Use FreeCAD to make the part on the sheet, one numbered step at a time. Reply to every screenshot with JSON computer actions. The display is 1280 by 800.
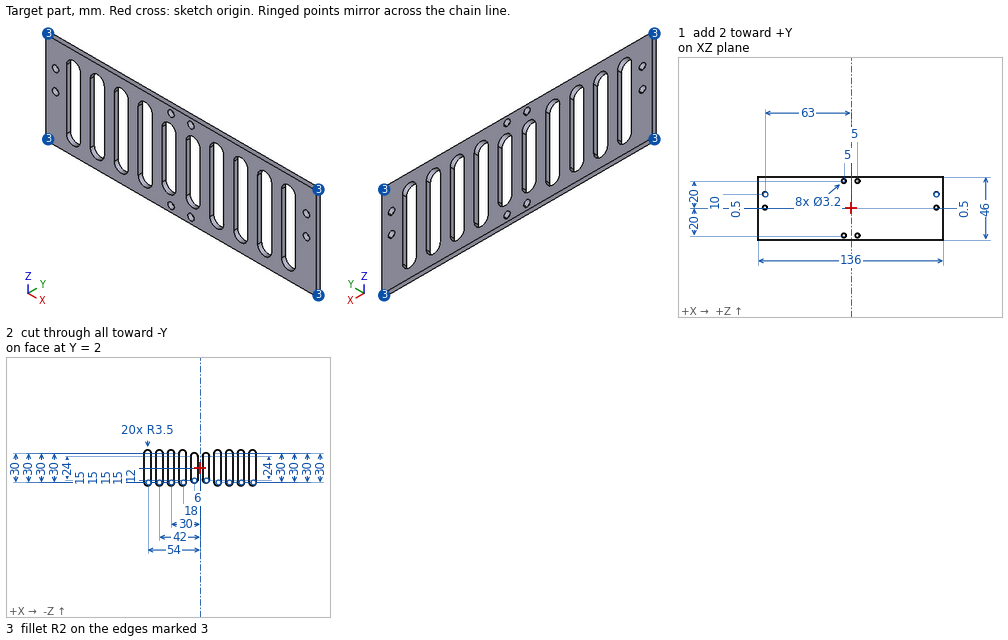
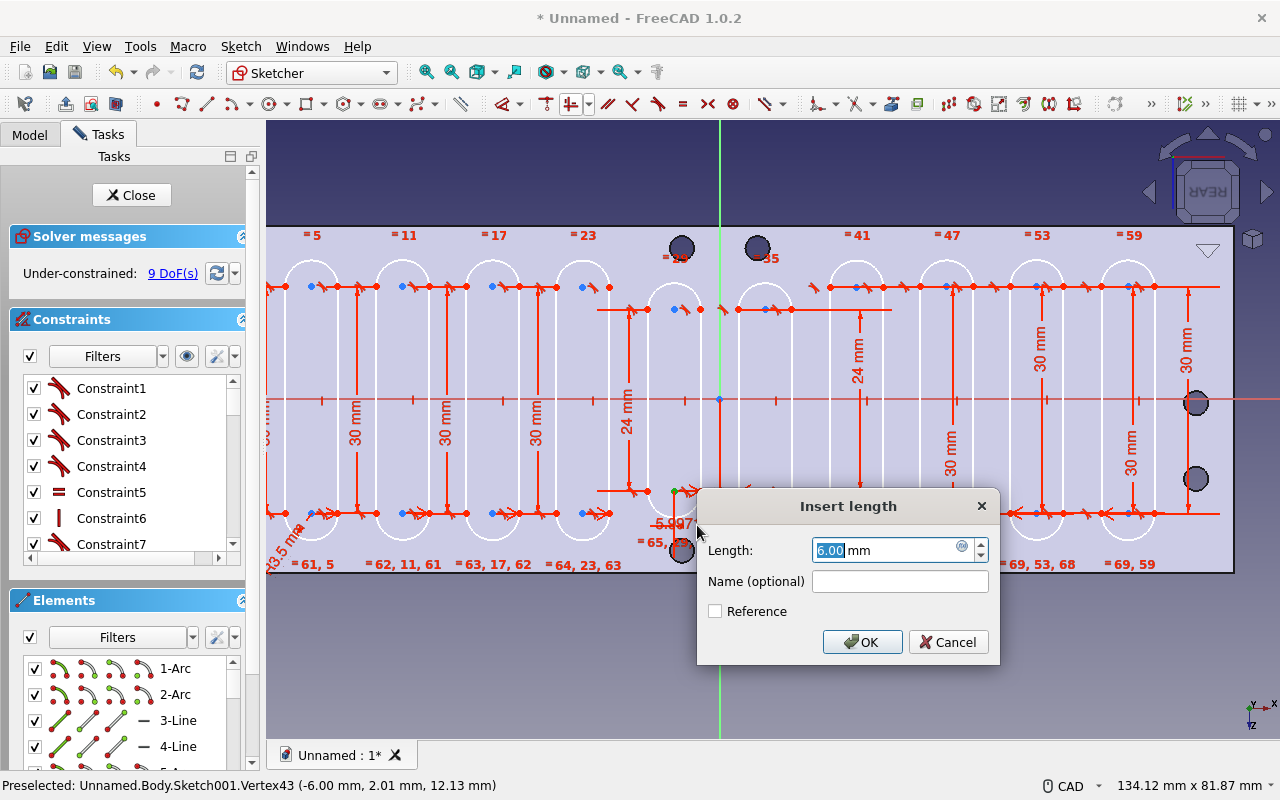
{"action": "type", "text": "6"}
{"action": "key", "text": "Return"}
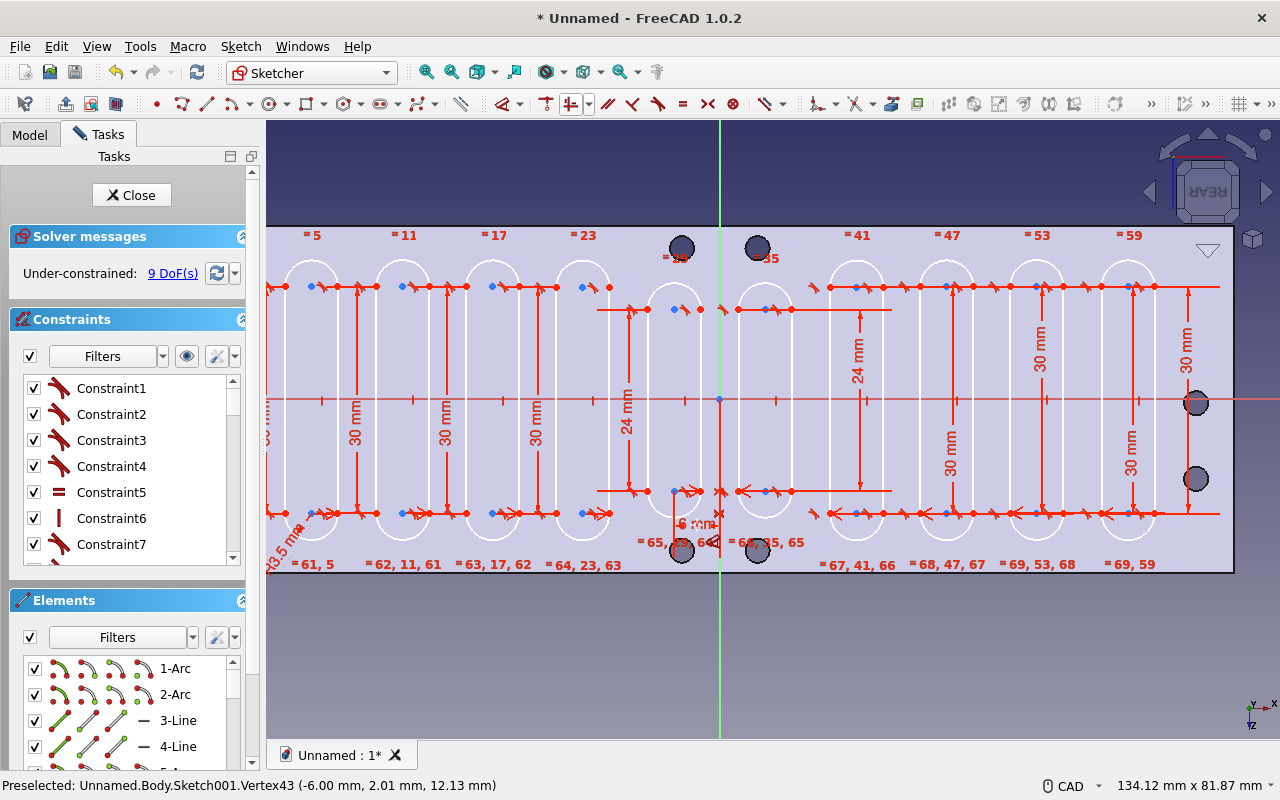
{"action": "scroll", "coordinate": [673, 491], "scroll_direction": "down", "scroll_amount": 2}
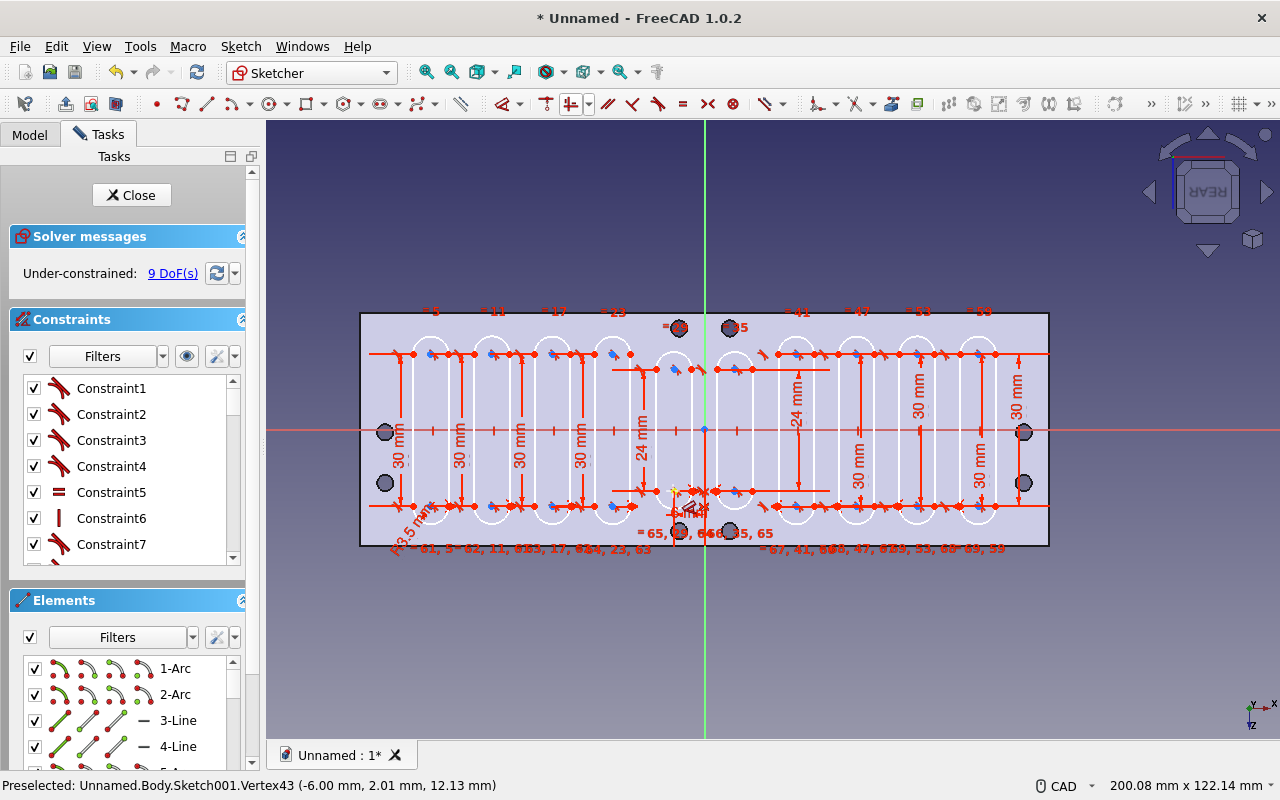
{"action": "left_click", "coordinate": [413, 506]}
{"action": "left_click", "coordinate": [379, 468]}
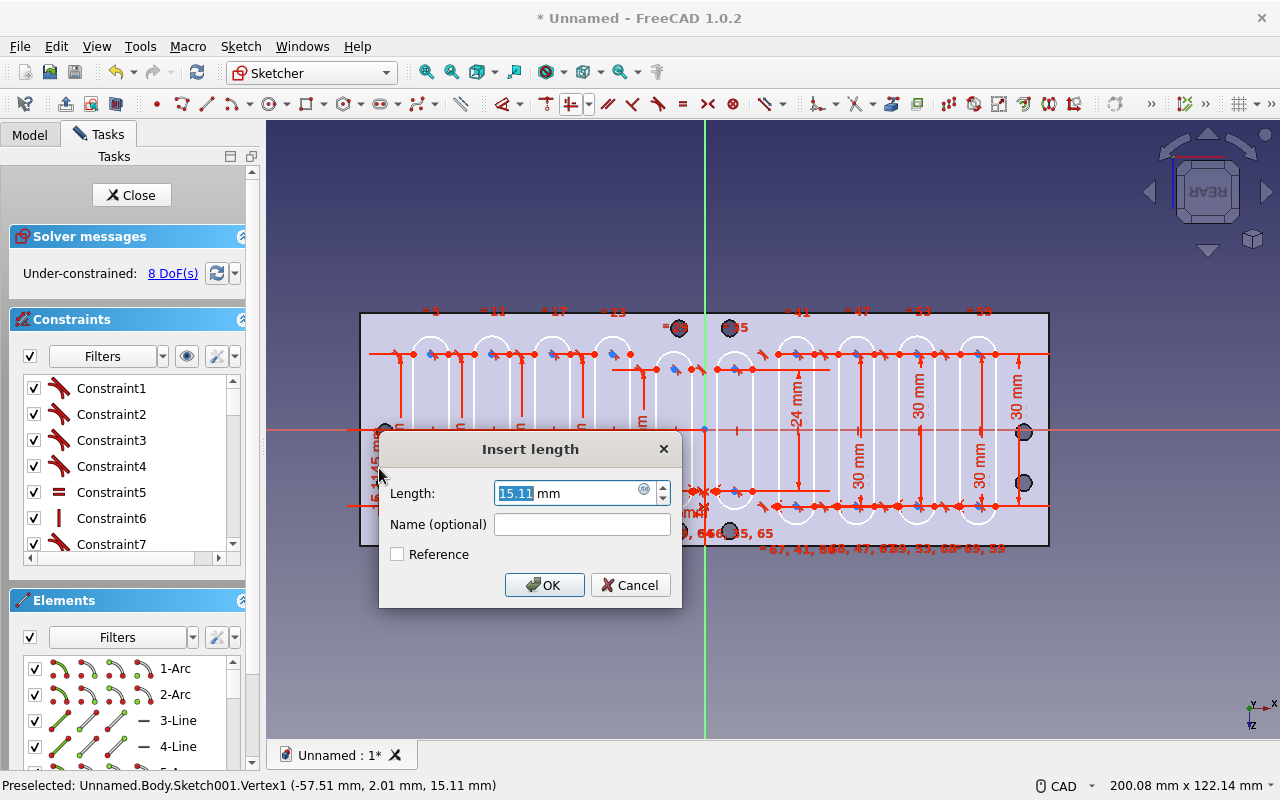
{"action": "type", "text": "15"}
{"action": "key", "text": "Return"}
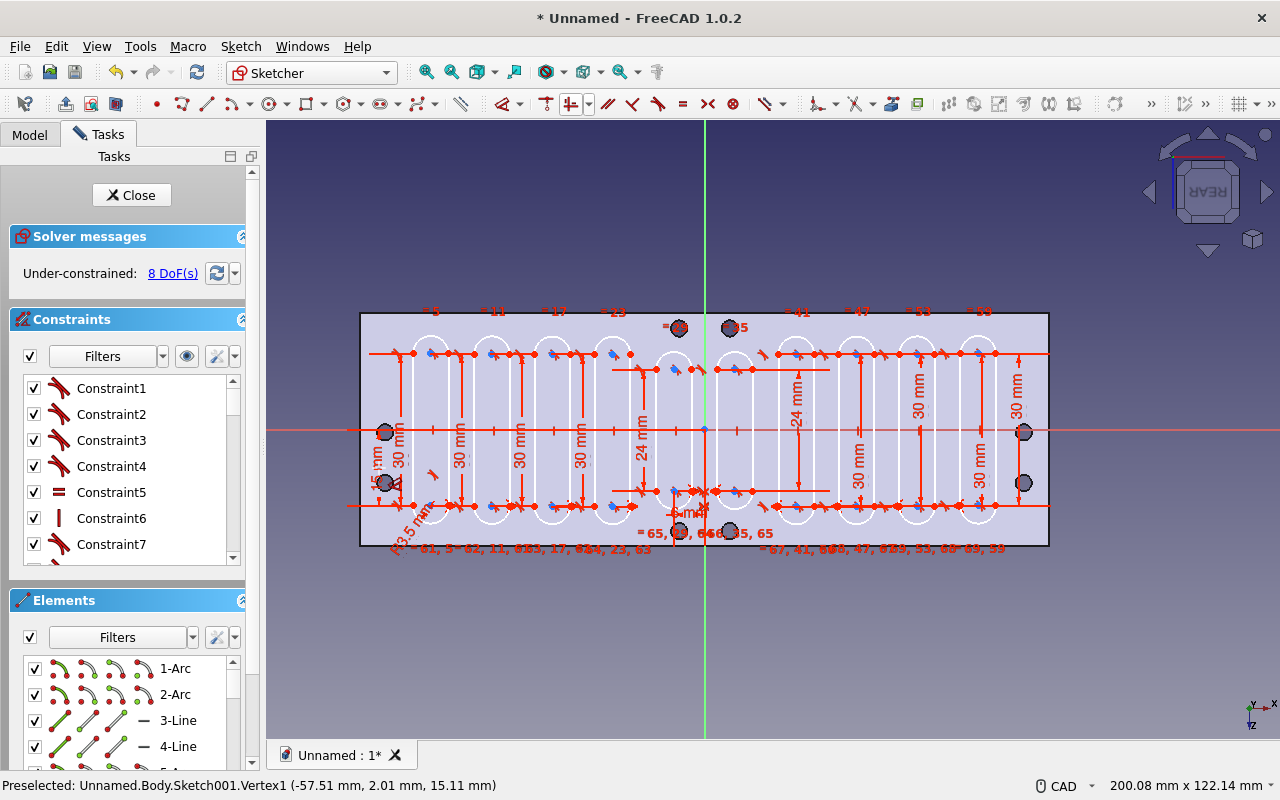
{"action": "left_click", "coordinate": [474, 506]}
{"action": "left_click", "coordinate": [739, 468]}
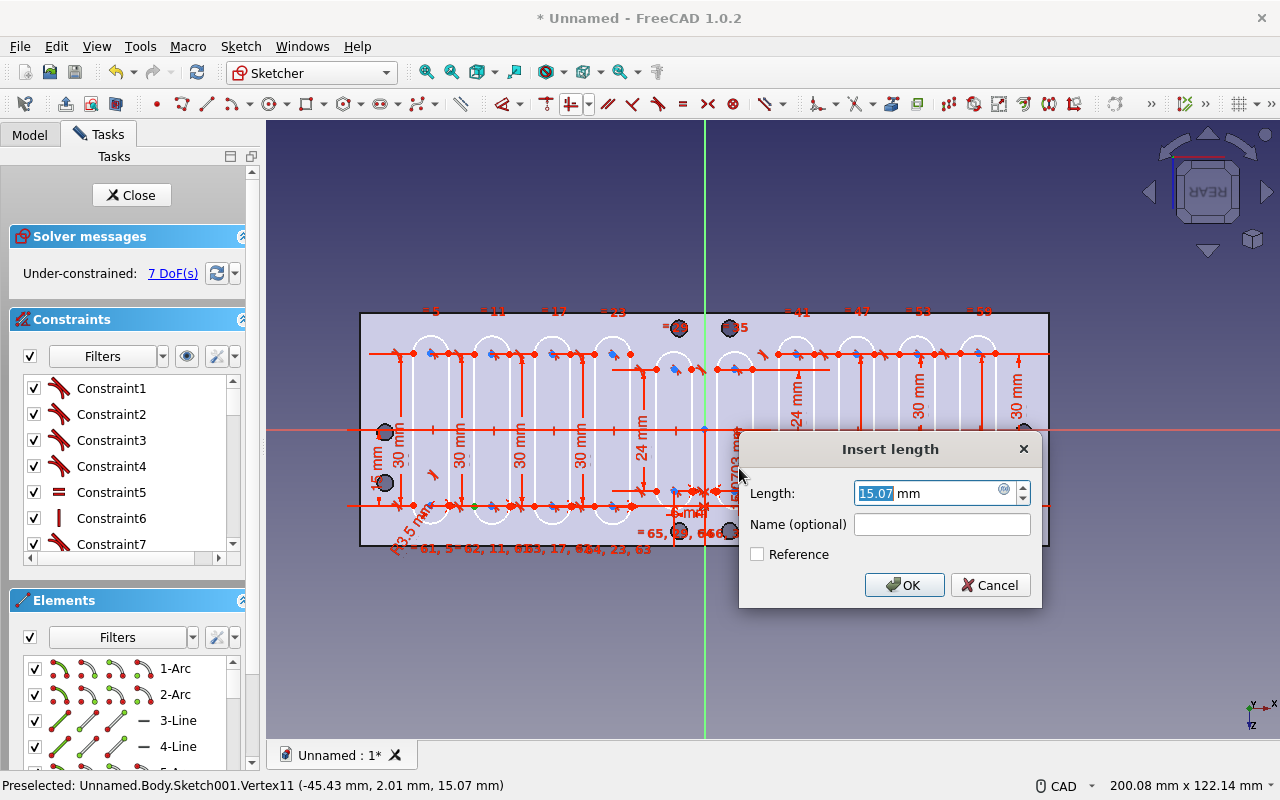
{"action": "type", "text": "15"}
{"action": "key", "text": "Return"}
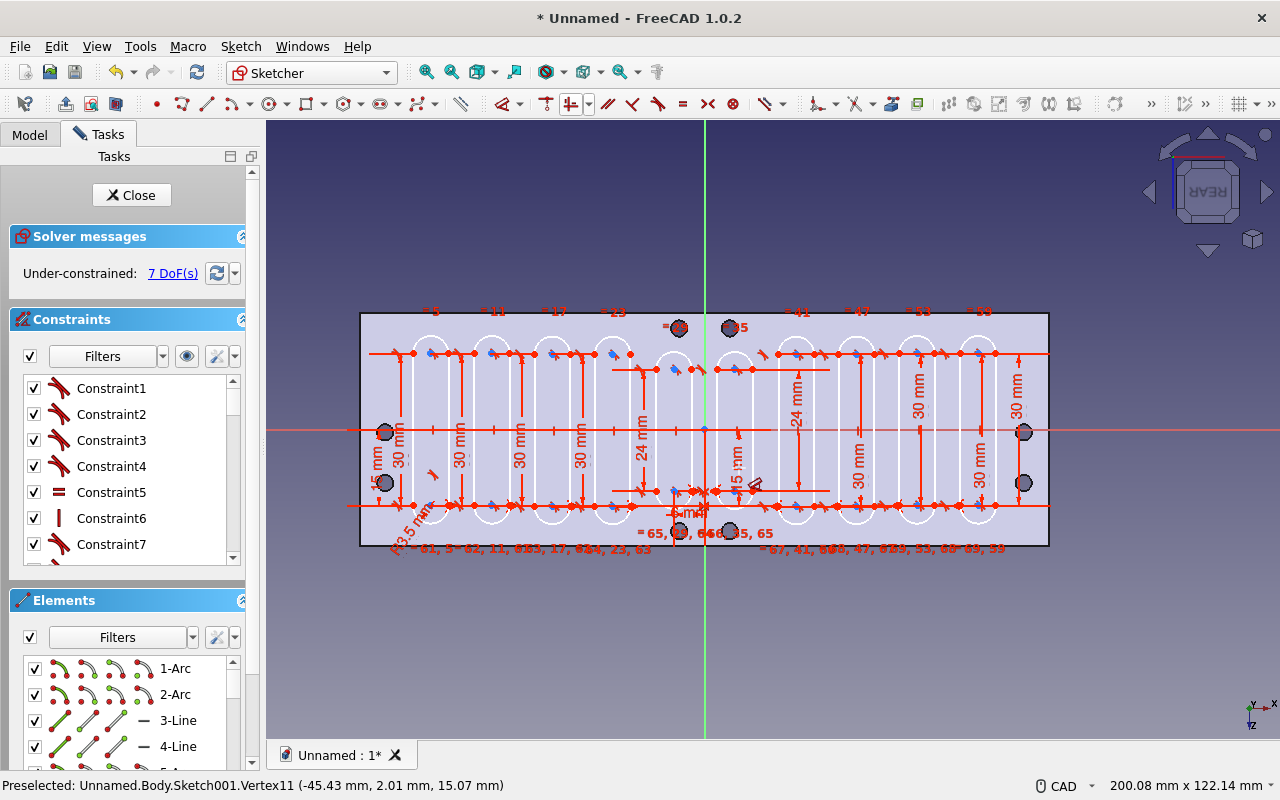
{"action": "left_click", "coordinate": [535, 506]}
{"action": "left_click", "coordinate": [429, 495]}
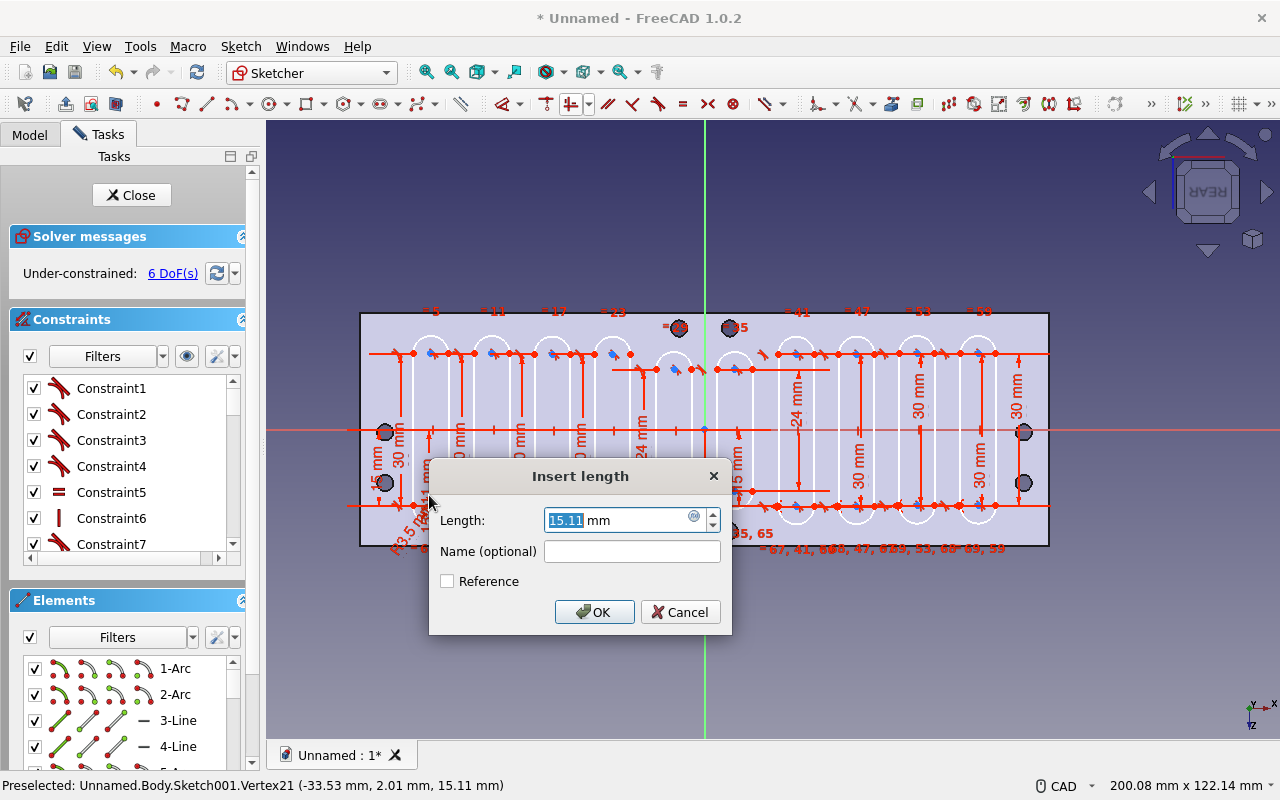
{"action": "type", "text": "15"}
{"action": "key", "text": "Return"}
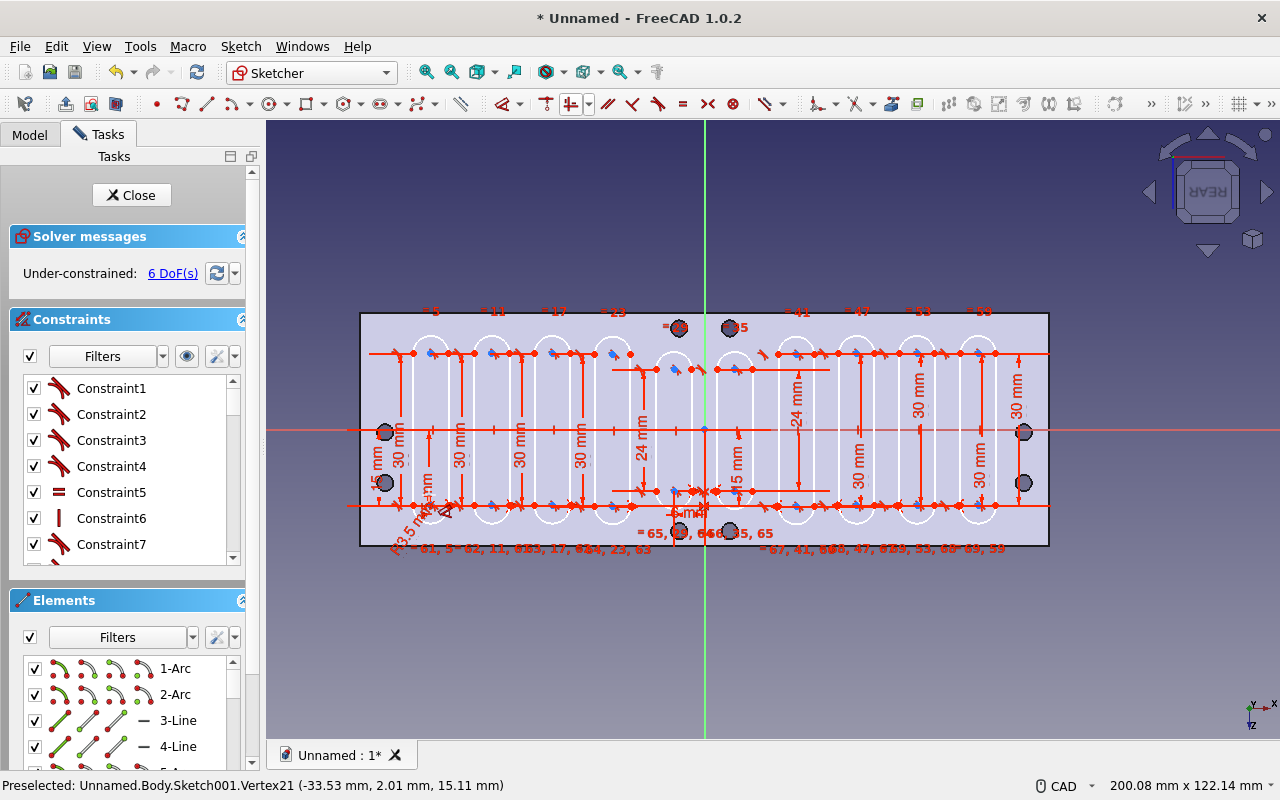
{"action": "left_click", "coordinate": [595, 507]}
{"action": "left_click", "coordinate": [489, 468]}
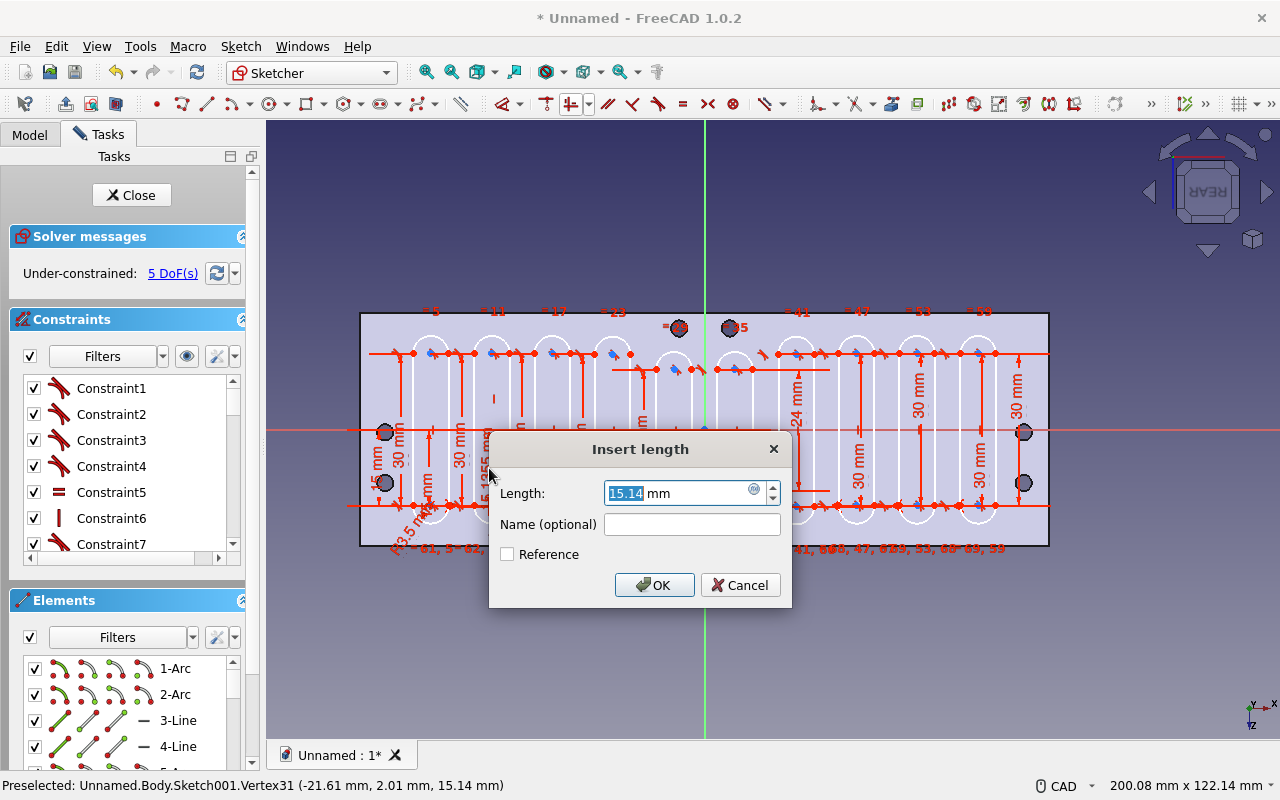
{"action": "type", "text": "15"}
{"action": "key", "text": "Return"}